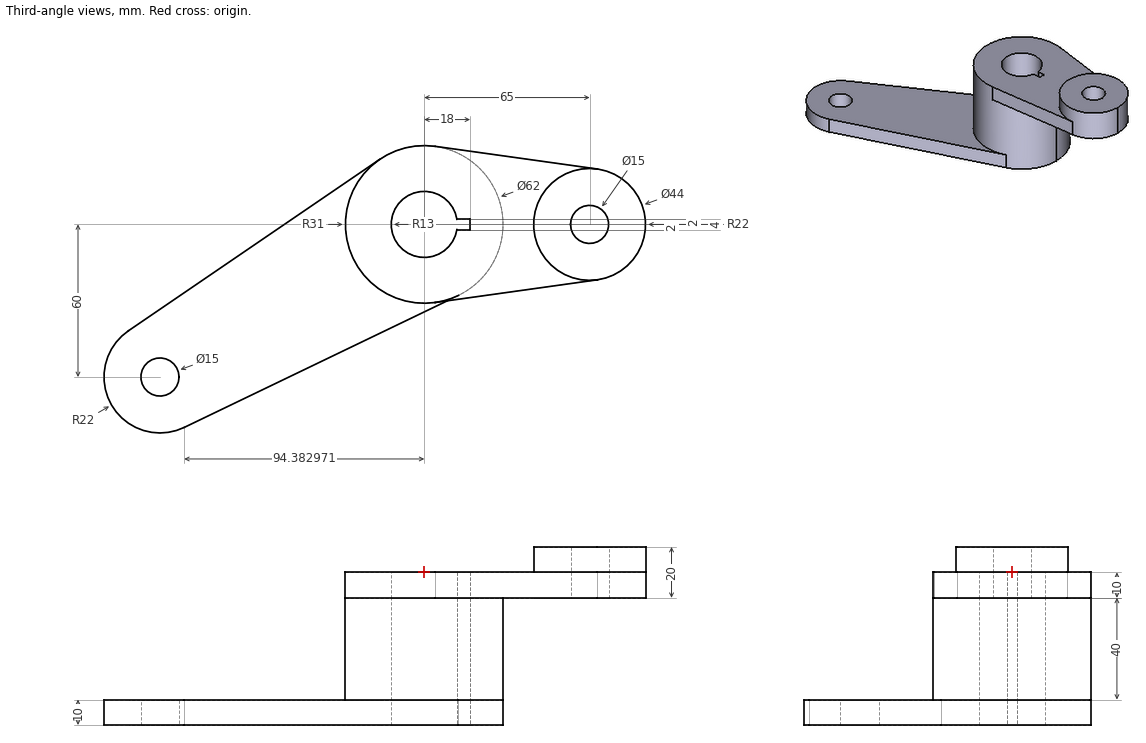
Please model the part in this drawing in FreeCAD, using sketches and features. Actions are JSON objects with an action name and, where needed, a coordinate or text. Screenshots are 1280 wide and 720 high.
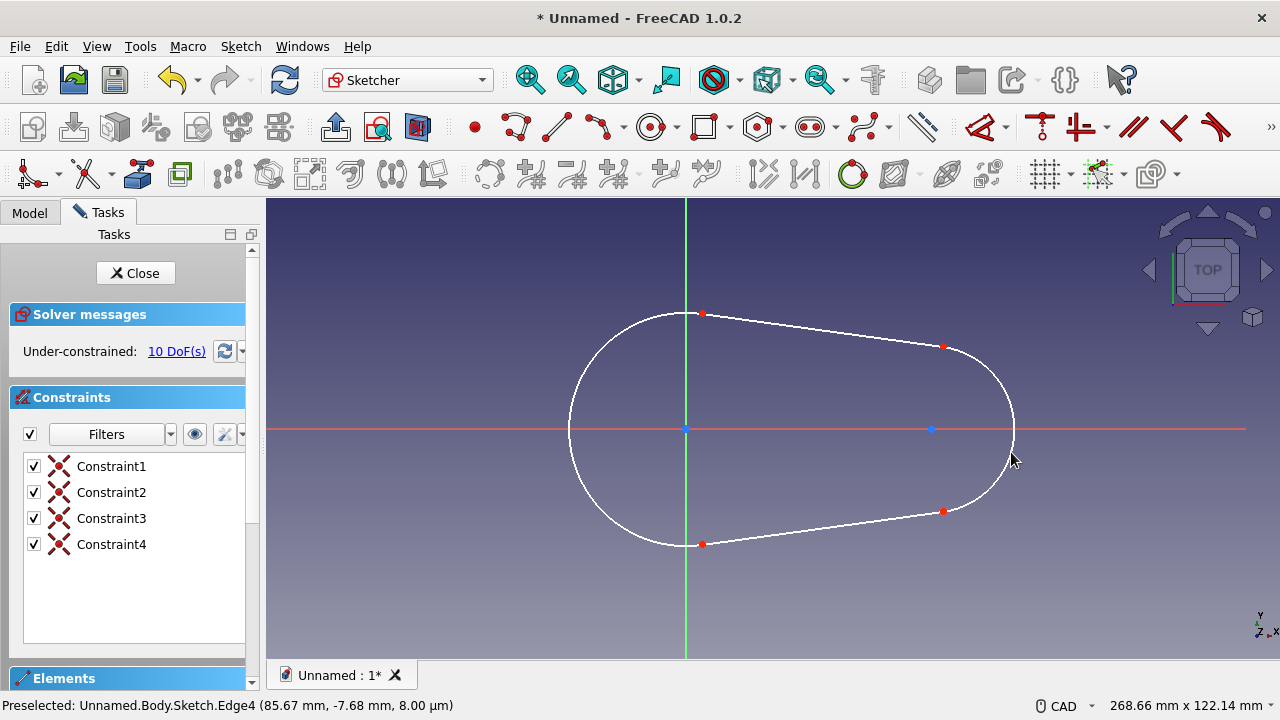
{"action": "left_click", "coordinate": [871, 337]}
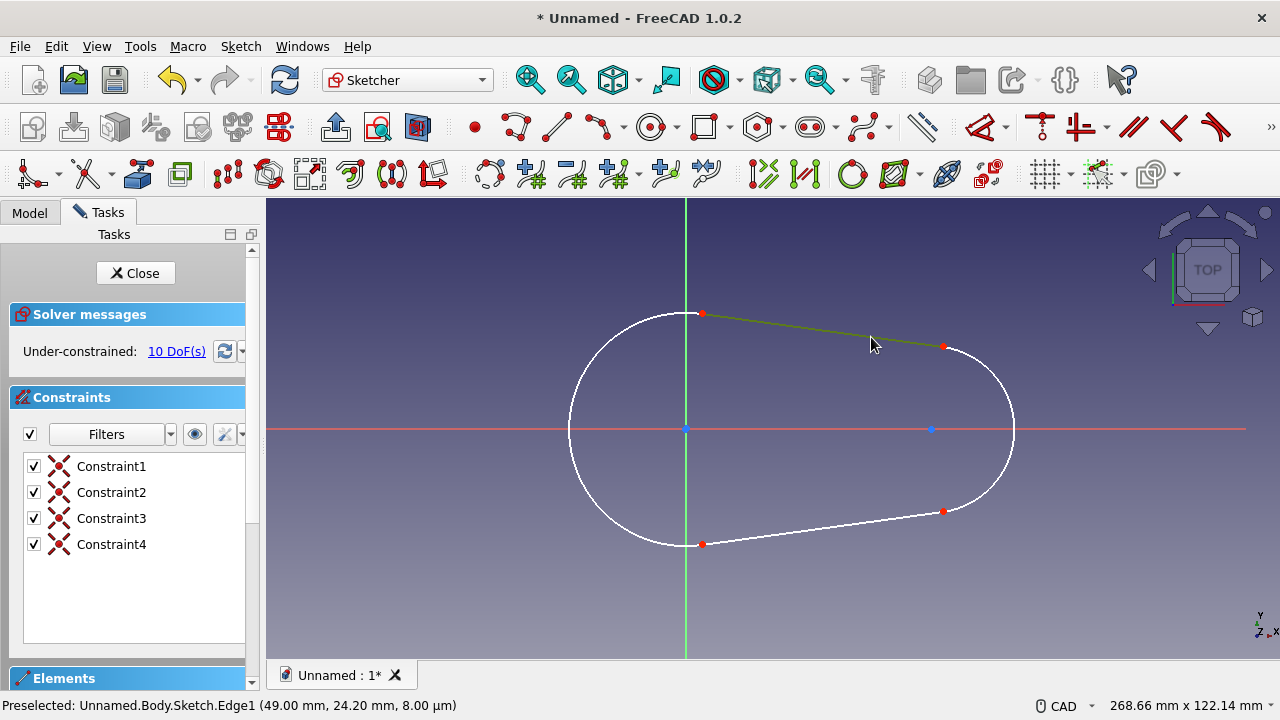
{"action": "left_click", "coordinate": [595, 356]}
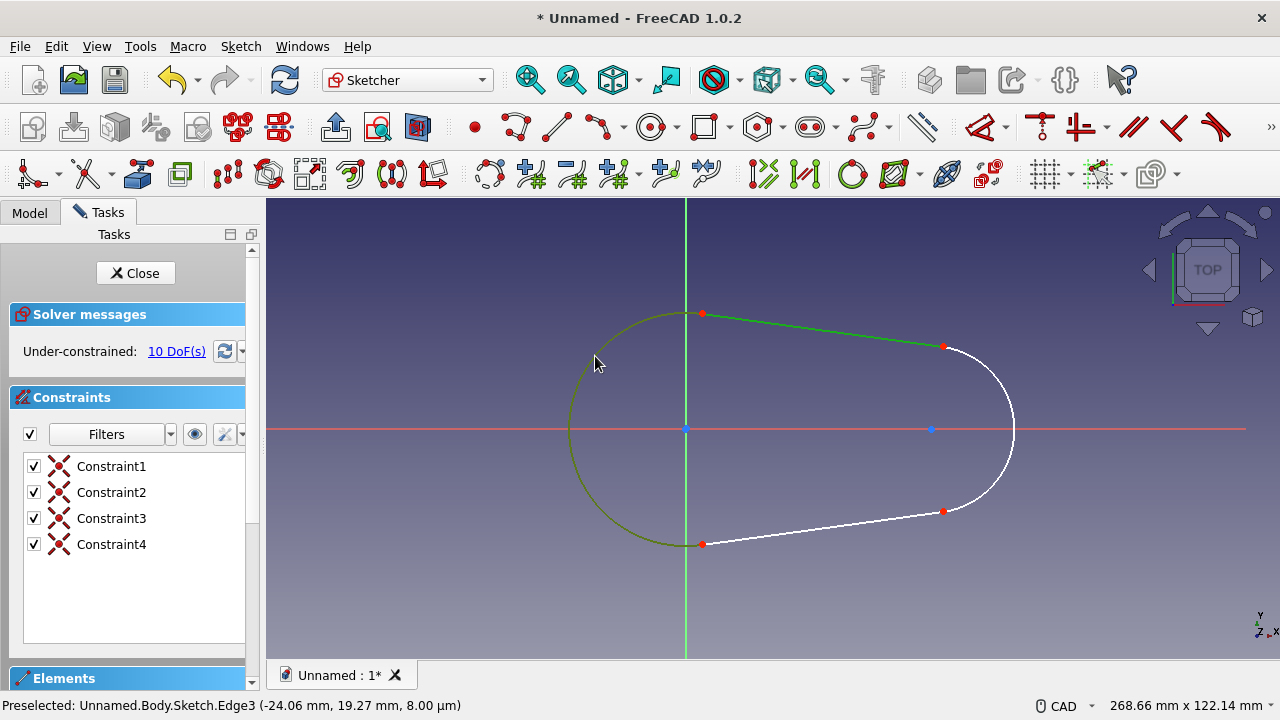
{"action": "key", "text": "t"}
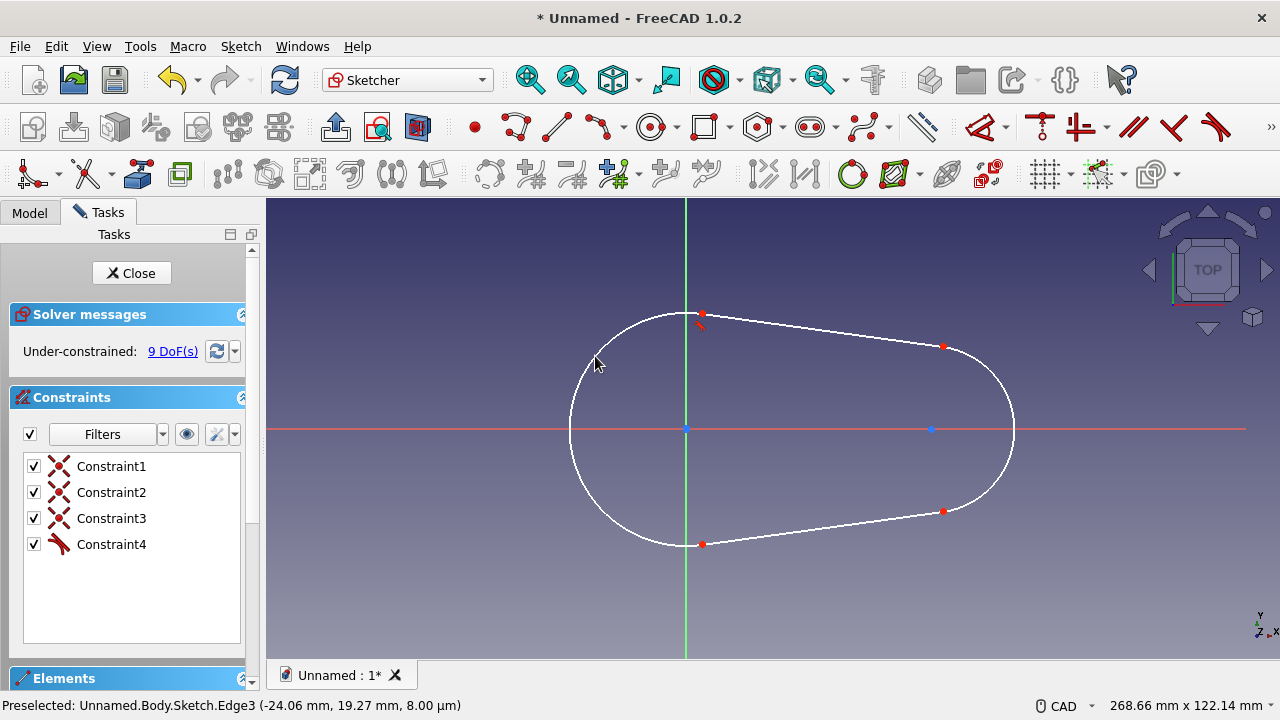
{"action": "left_click", "coordinate": [871, 337]}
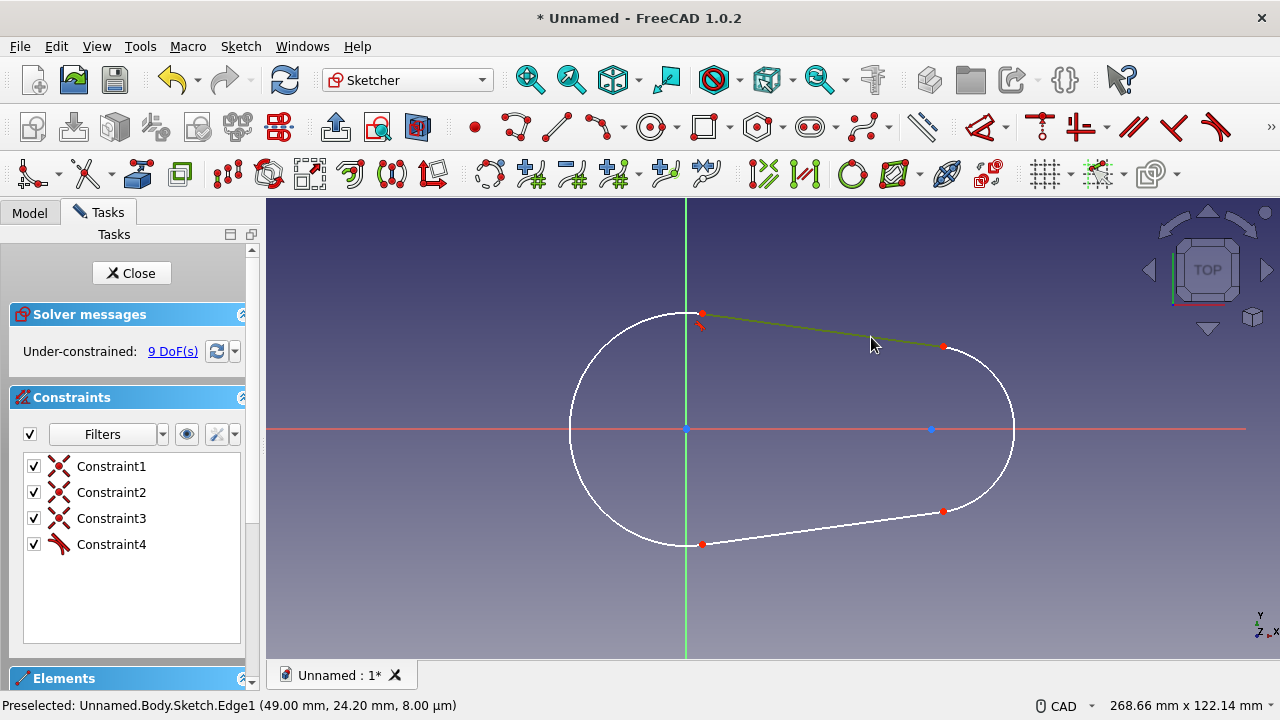
{"action": "left_click", "coordinate": [1001, 475]}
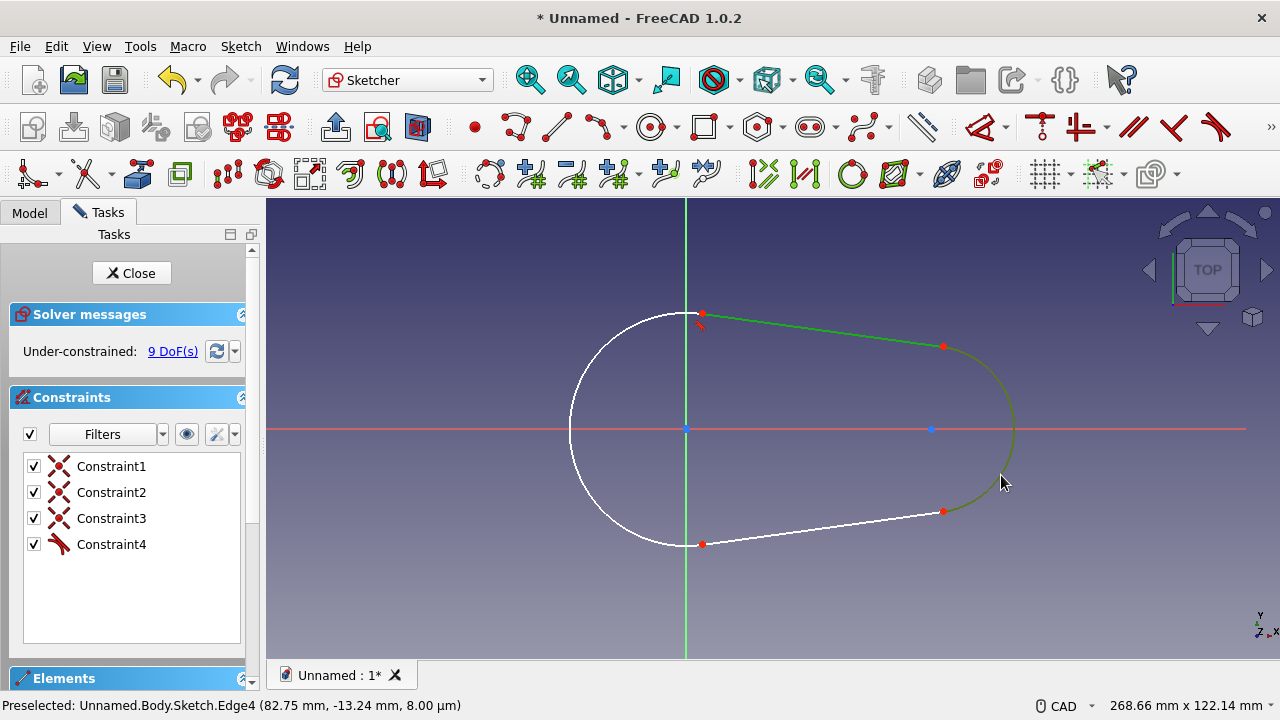
{"action": "key", "text": "t"}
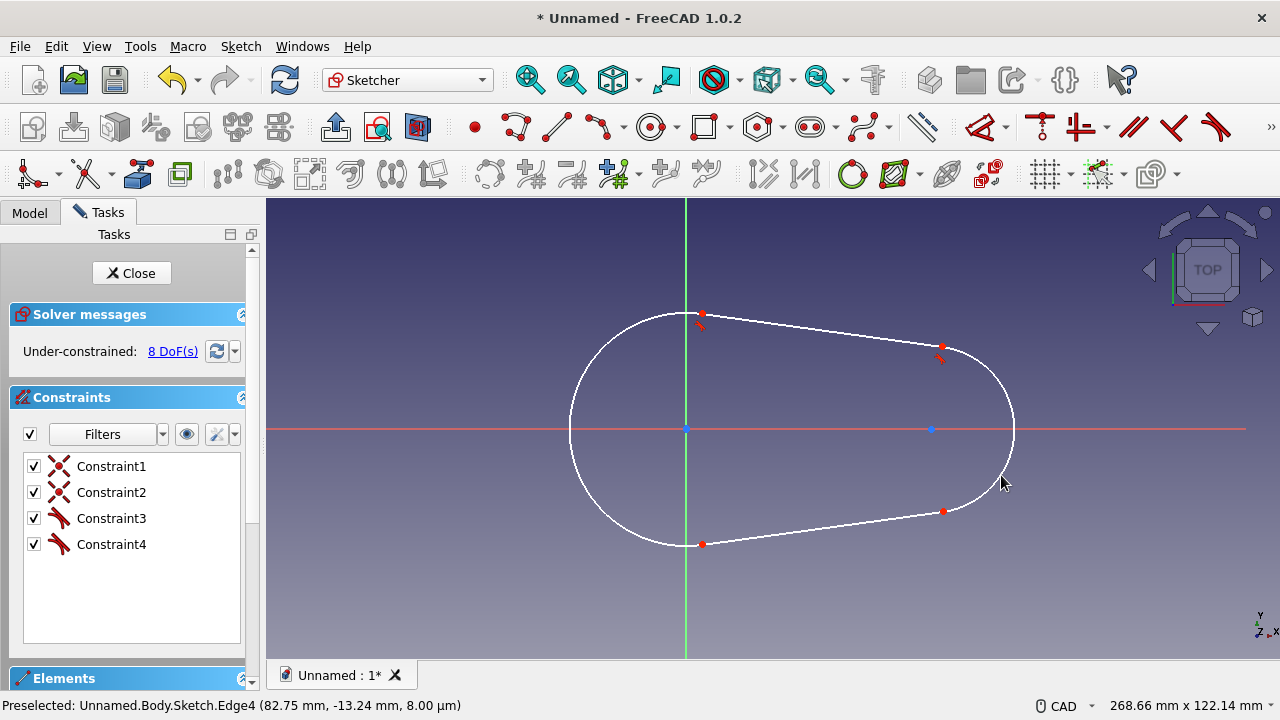
{"action": "left_click", "coordinate": [774, 535]}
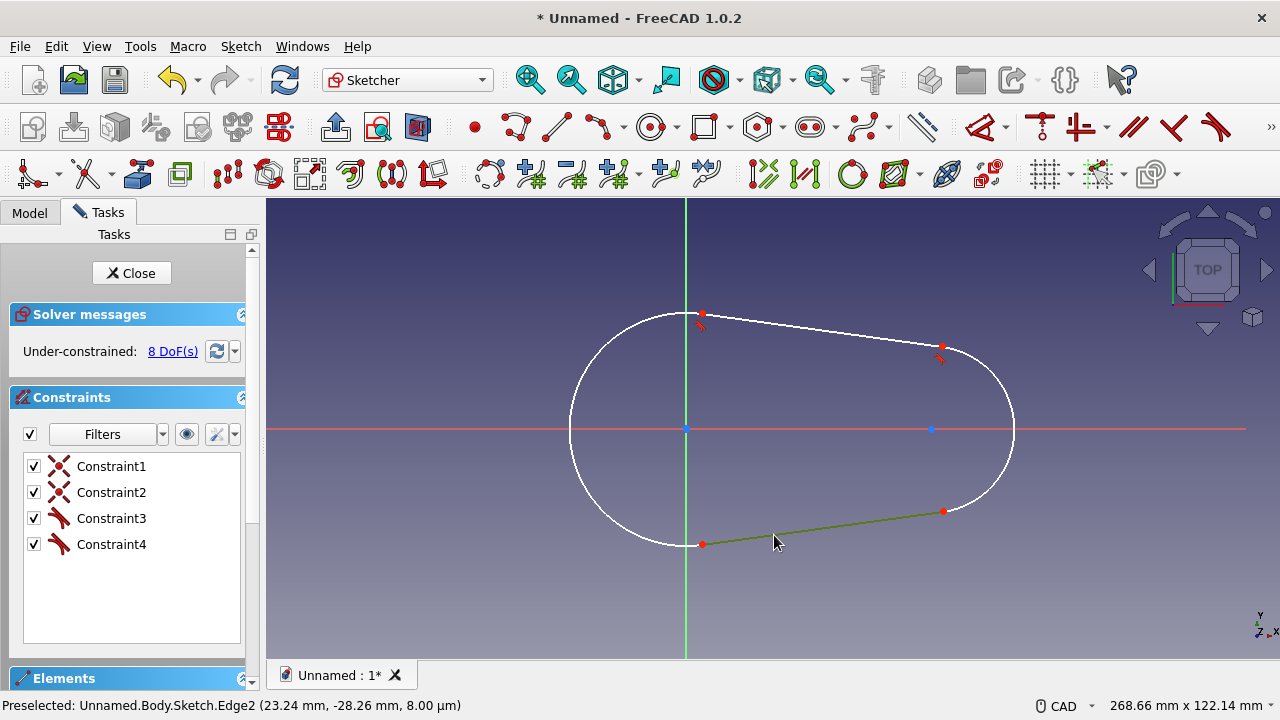
{"action": "left_click", "coordinate": [596, 356]}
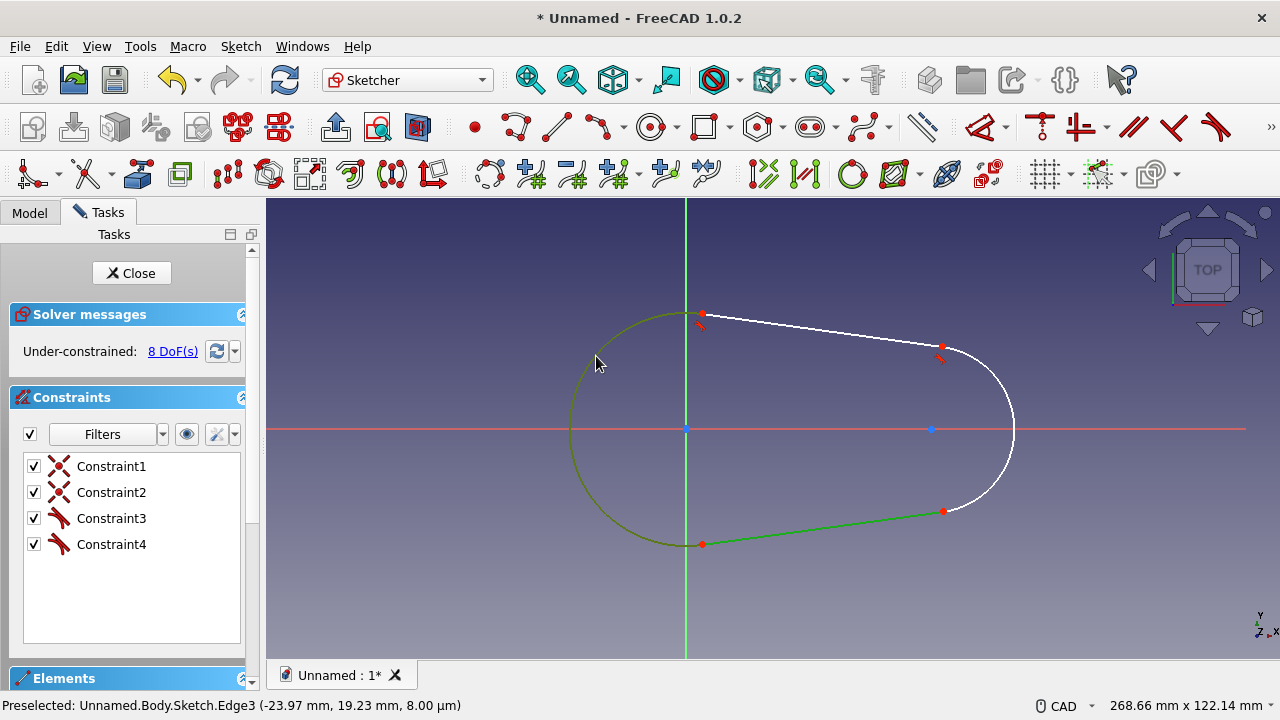
{"action": "key", "text": "t"}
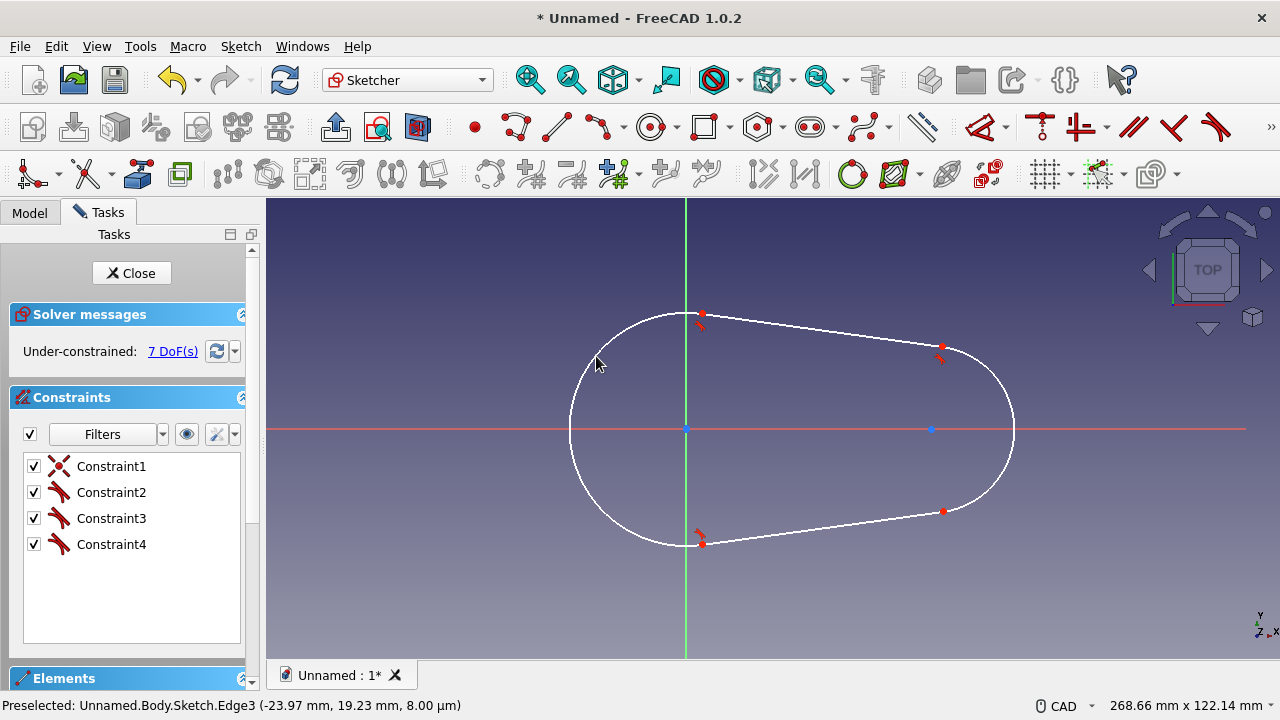
{"action": "left_click", "coordinate": [774, 535]}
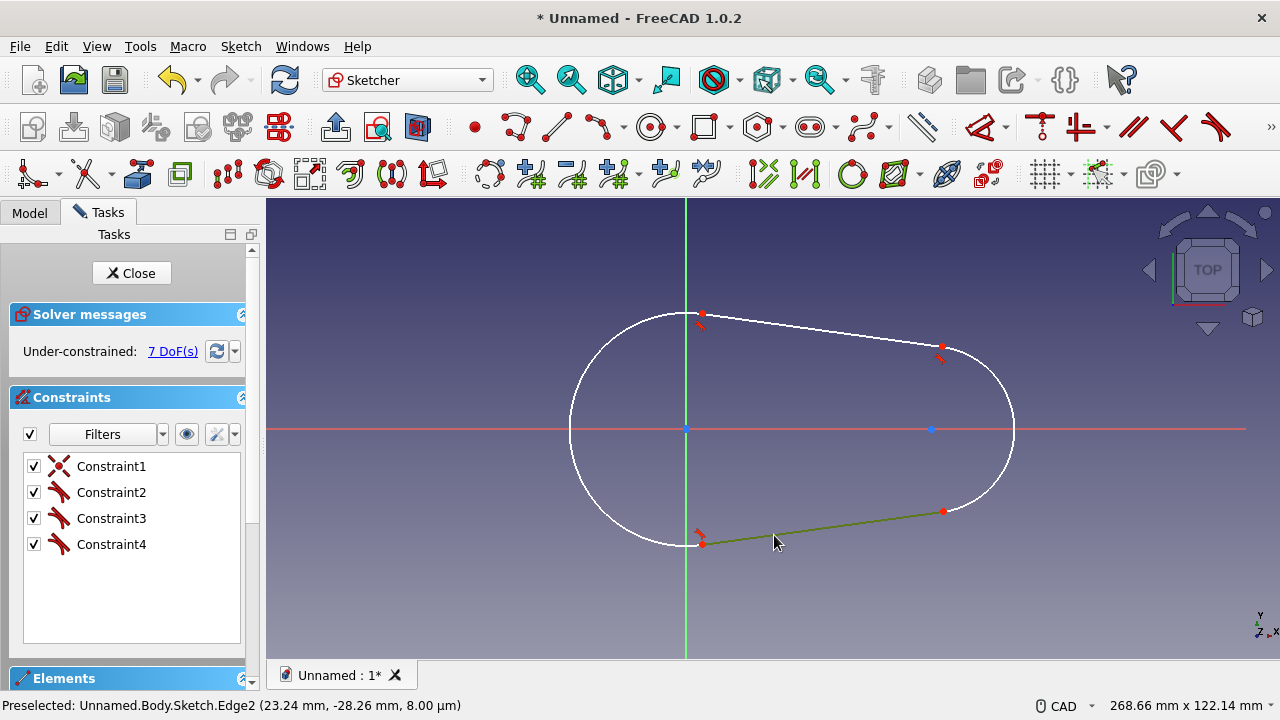
{"action": "left_click", "coordinate": [1001, 474]}